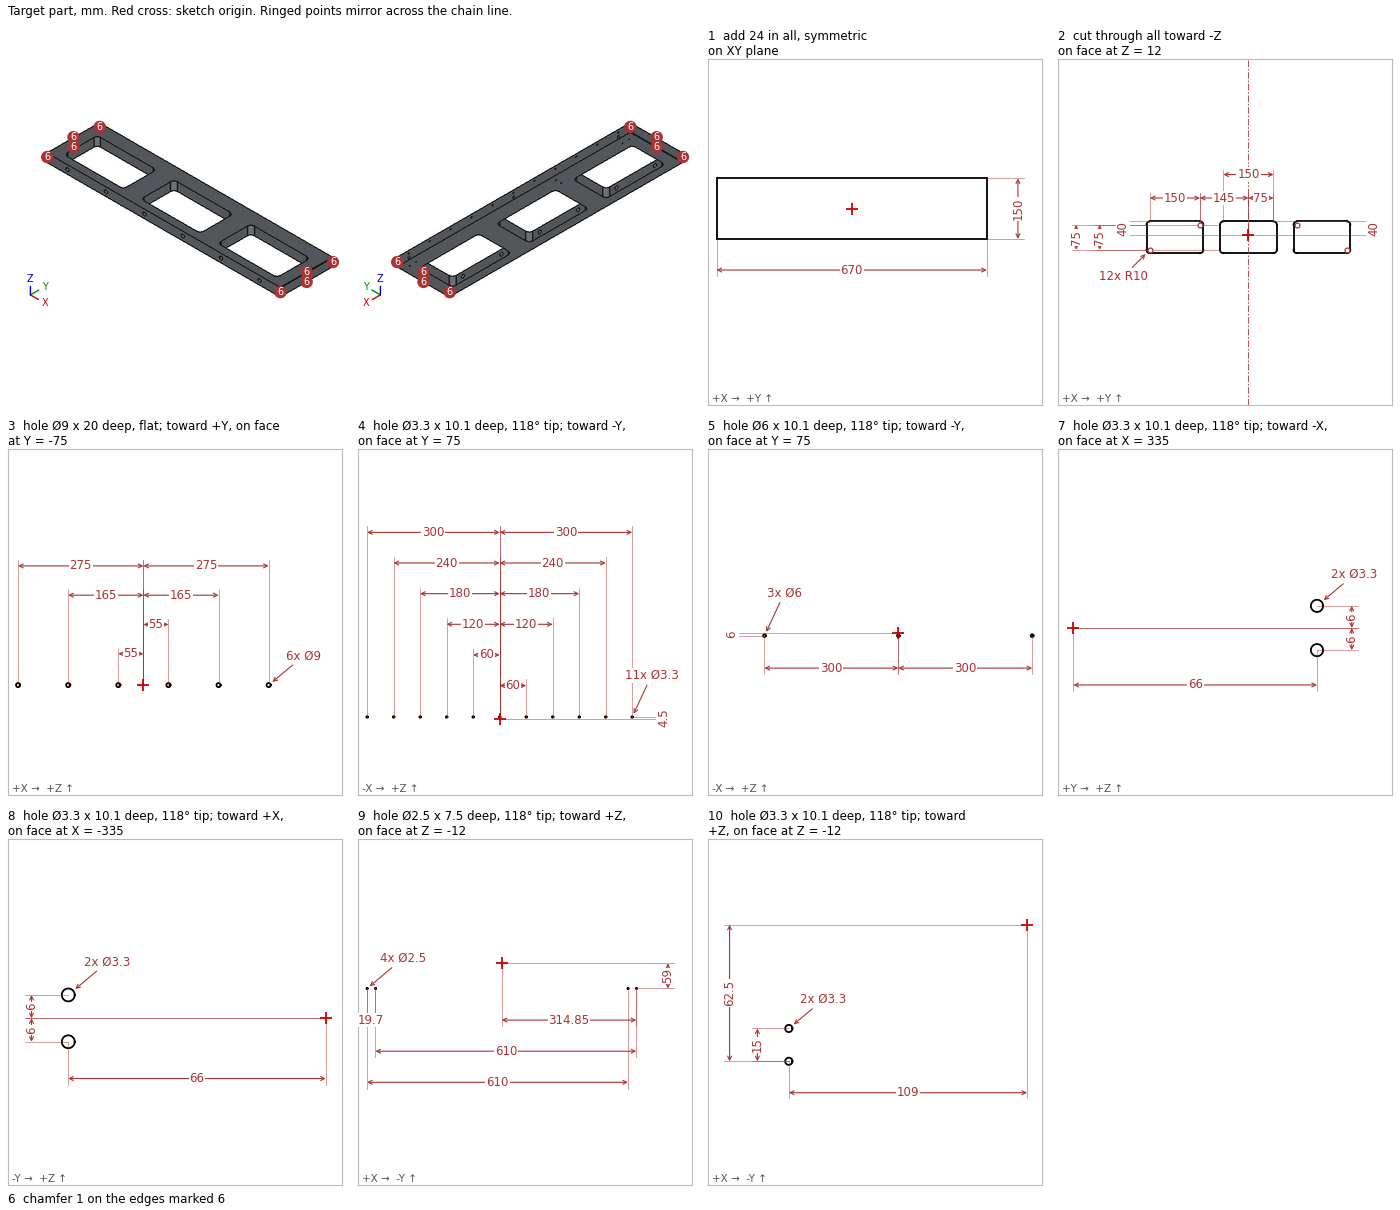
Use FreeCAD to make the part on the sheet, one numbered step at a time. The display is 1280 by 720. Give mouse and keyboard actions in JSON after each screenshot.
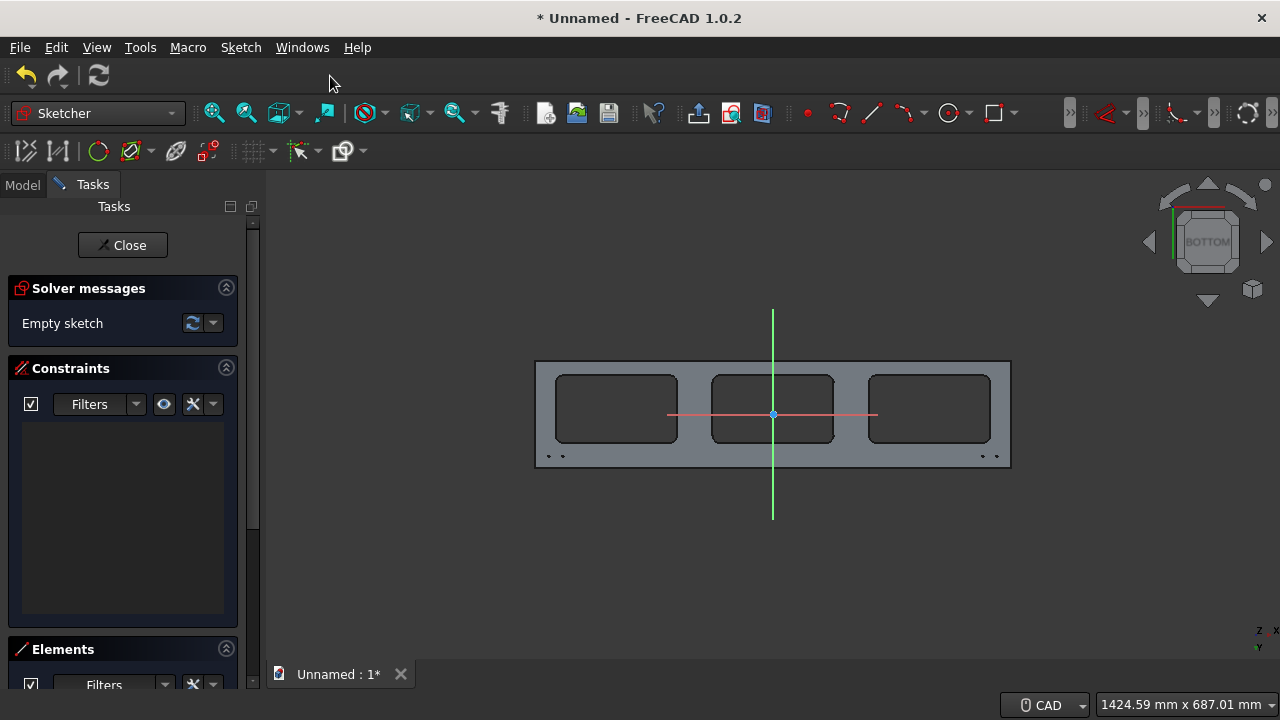
{"action": "scroll", "coordinate": [695, 456], "scroll_direction": "up", "scroll_amount": 15}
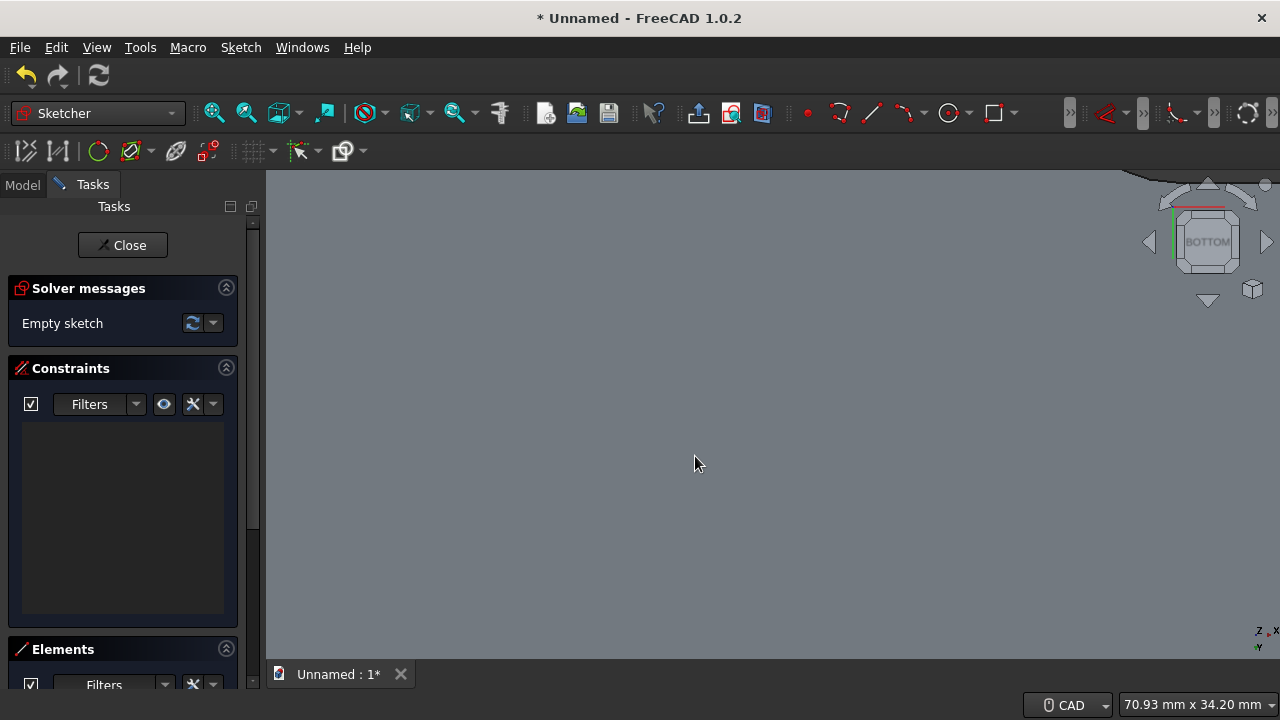
{"action": "left_click", "coordinate": [950, 114]}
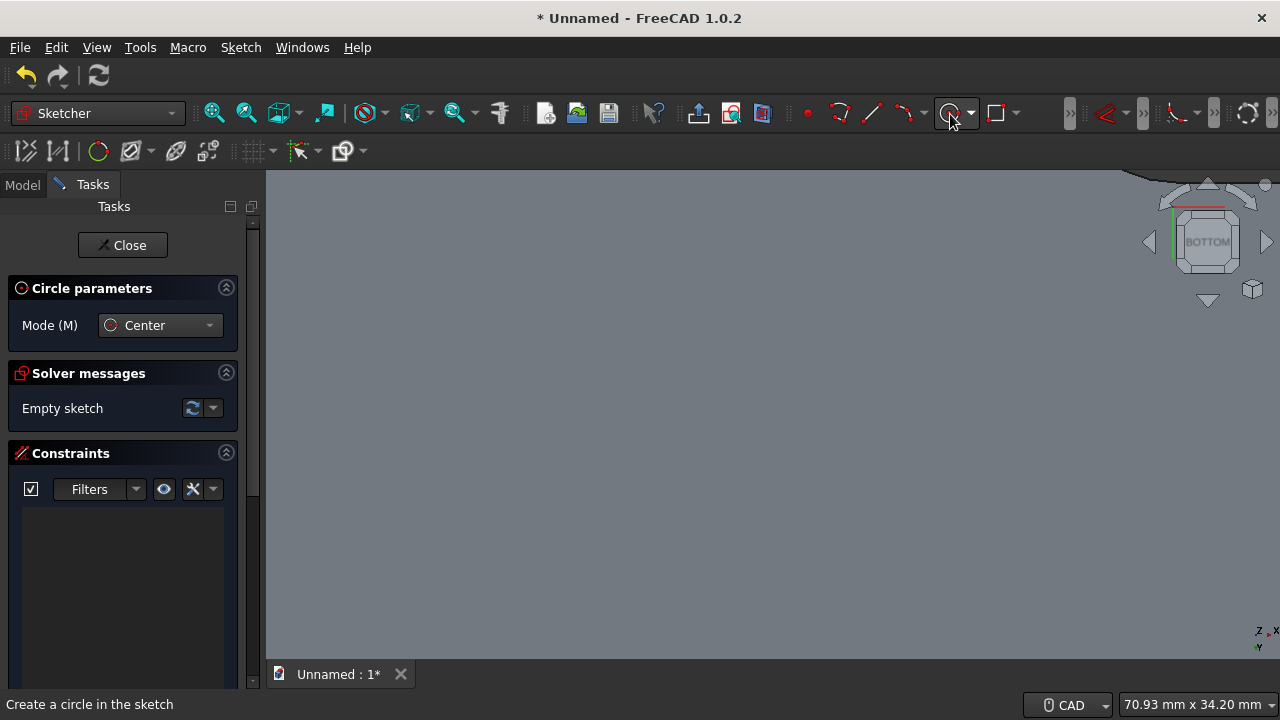
{"action": "left_click", "coordinate": [695, 505]}
{"action": "mouse_move", "coordinate": [712, 488]}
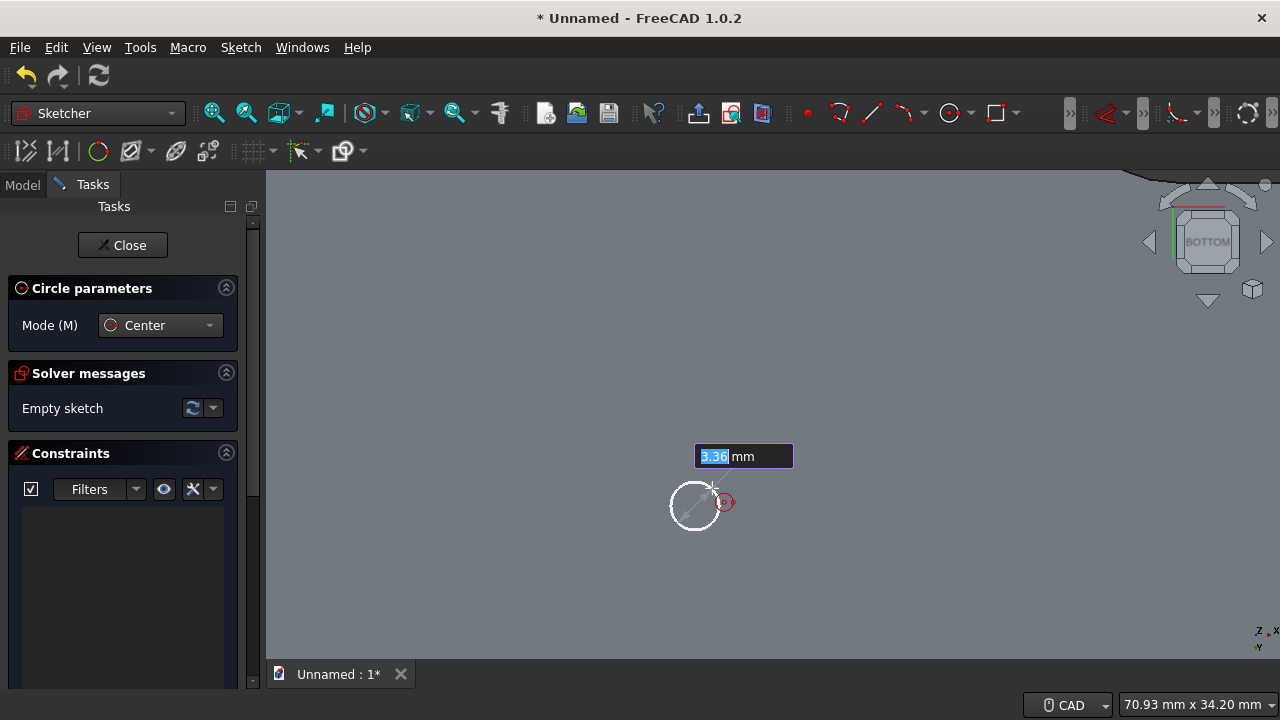
{"action": "type", "text": "3.3"}
{"action": "key", "text": "Return"}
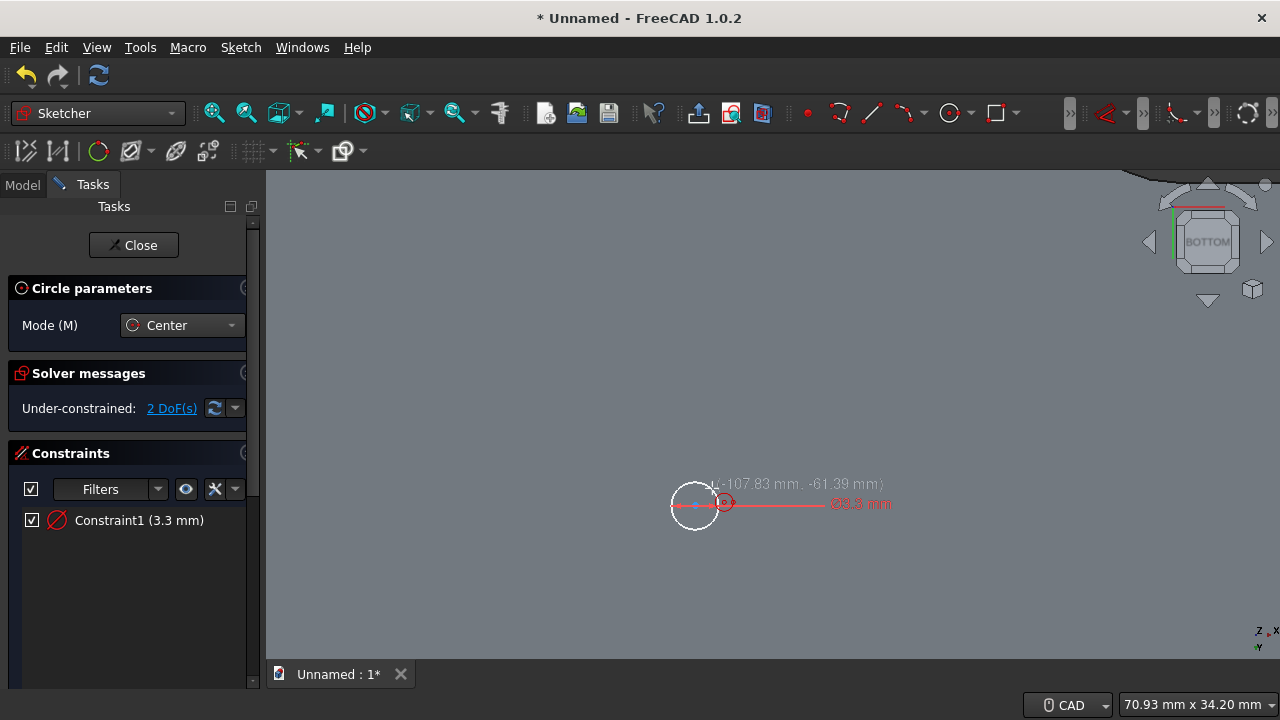
{"action": "left_click", "coordinate": [695, 290]}
{"action": "mouse_move", "coordinate": [712, 274]}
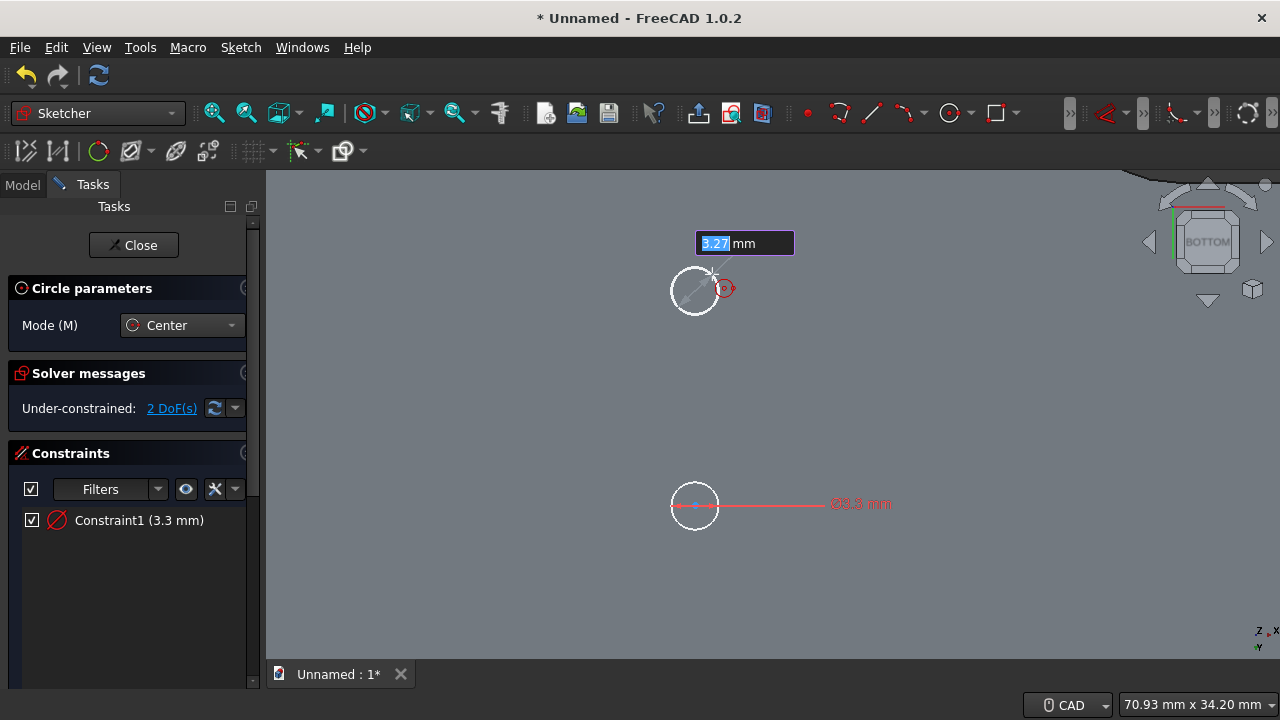
{"action": "type", "text": "3.3"}
{"action": "key", "text": "Return"}
{"action": "key", "text": "Escape"}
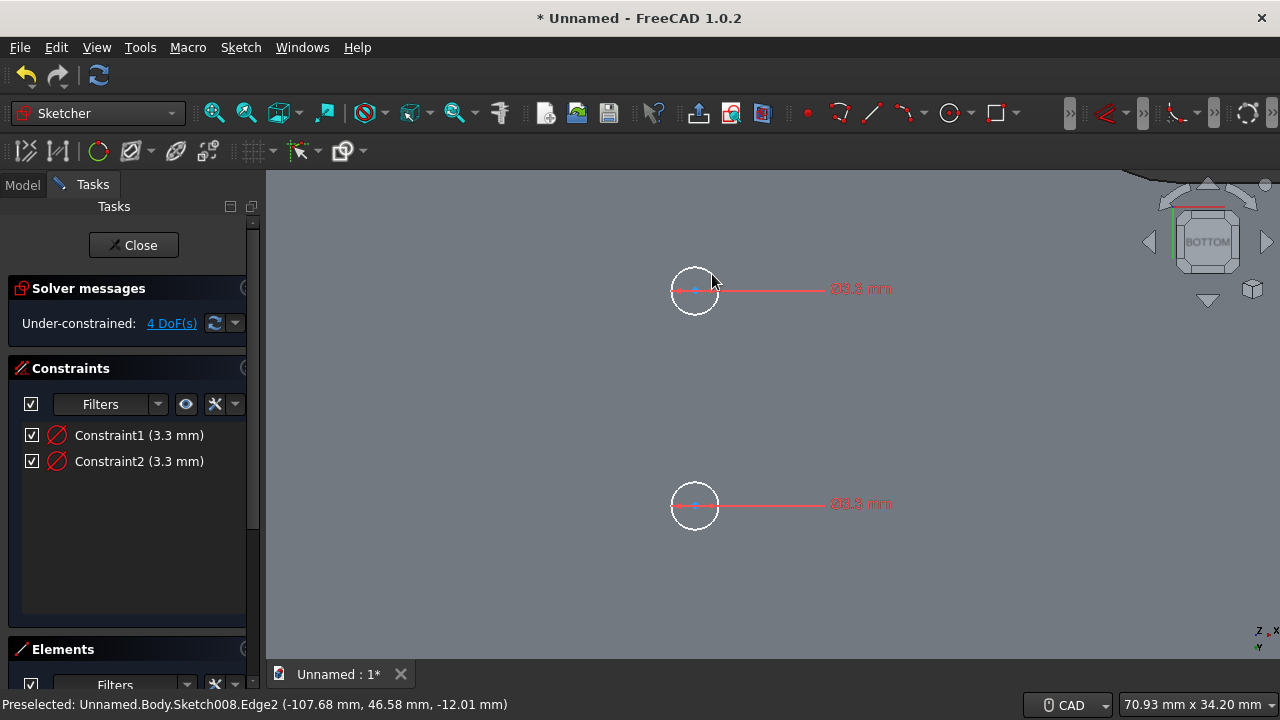
{"action": "left_click", "coordinate": [695, 506]}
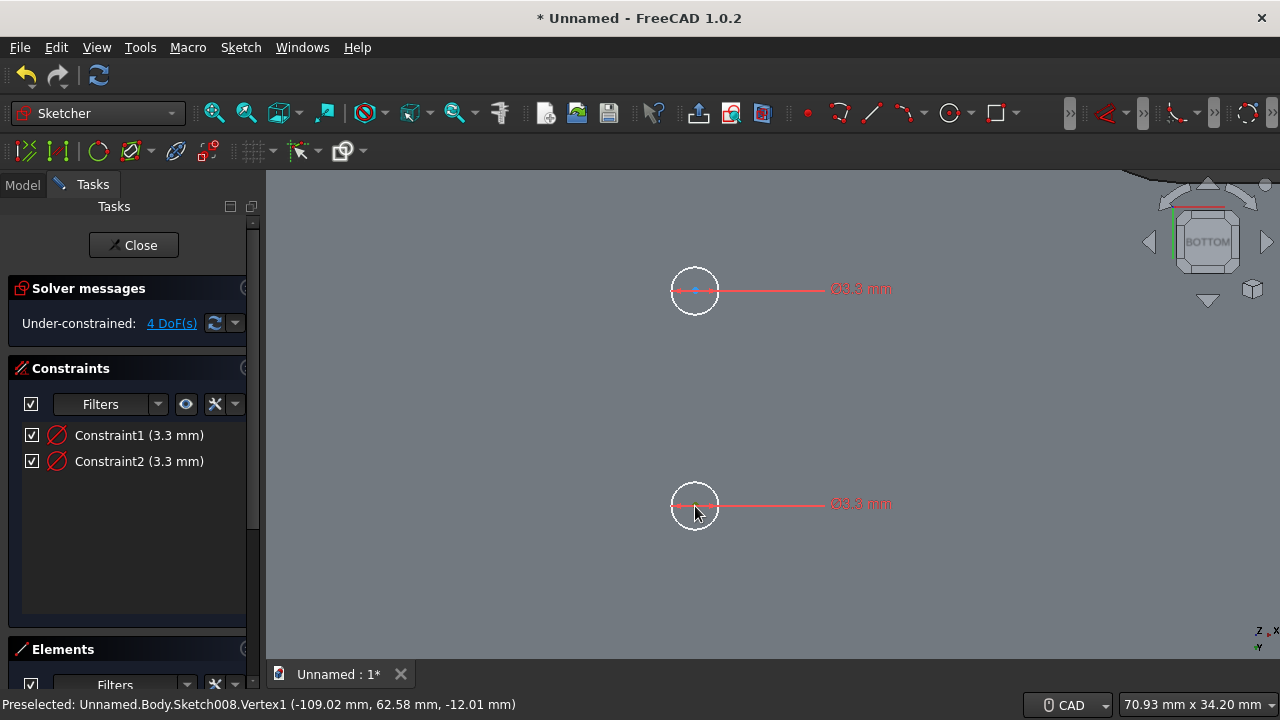
{"action": "left_click", "coordinate": [695, 291]}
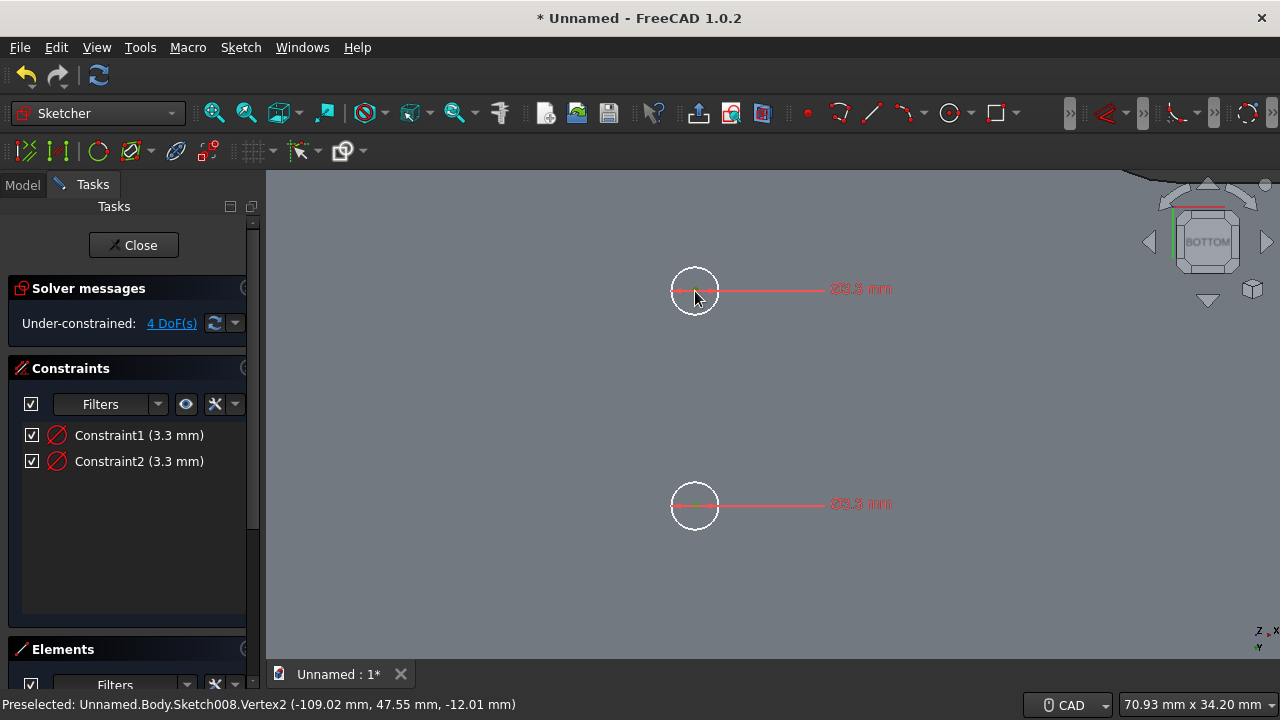
{"action": "key", "text": "v"}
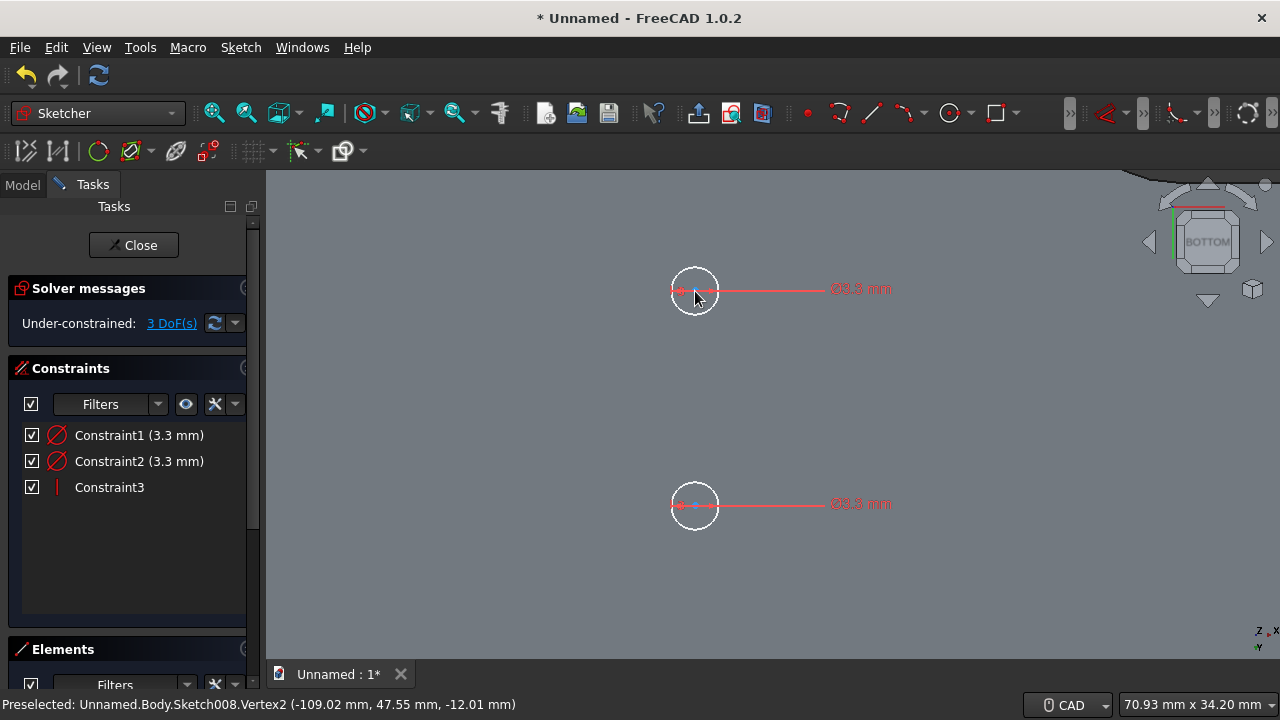
{"action": "left_click", "coordinate": [1106, 114]}